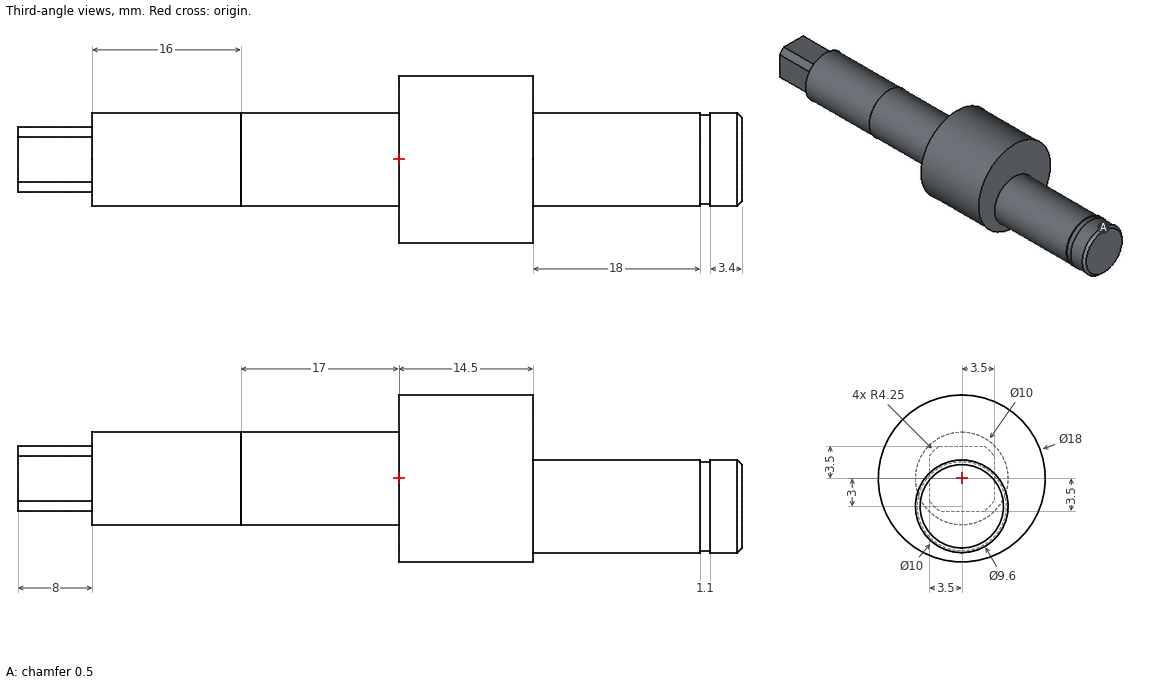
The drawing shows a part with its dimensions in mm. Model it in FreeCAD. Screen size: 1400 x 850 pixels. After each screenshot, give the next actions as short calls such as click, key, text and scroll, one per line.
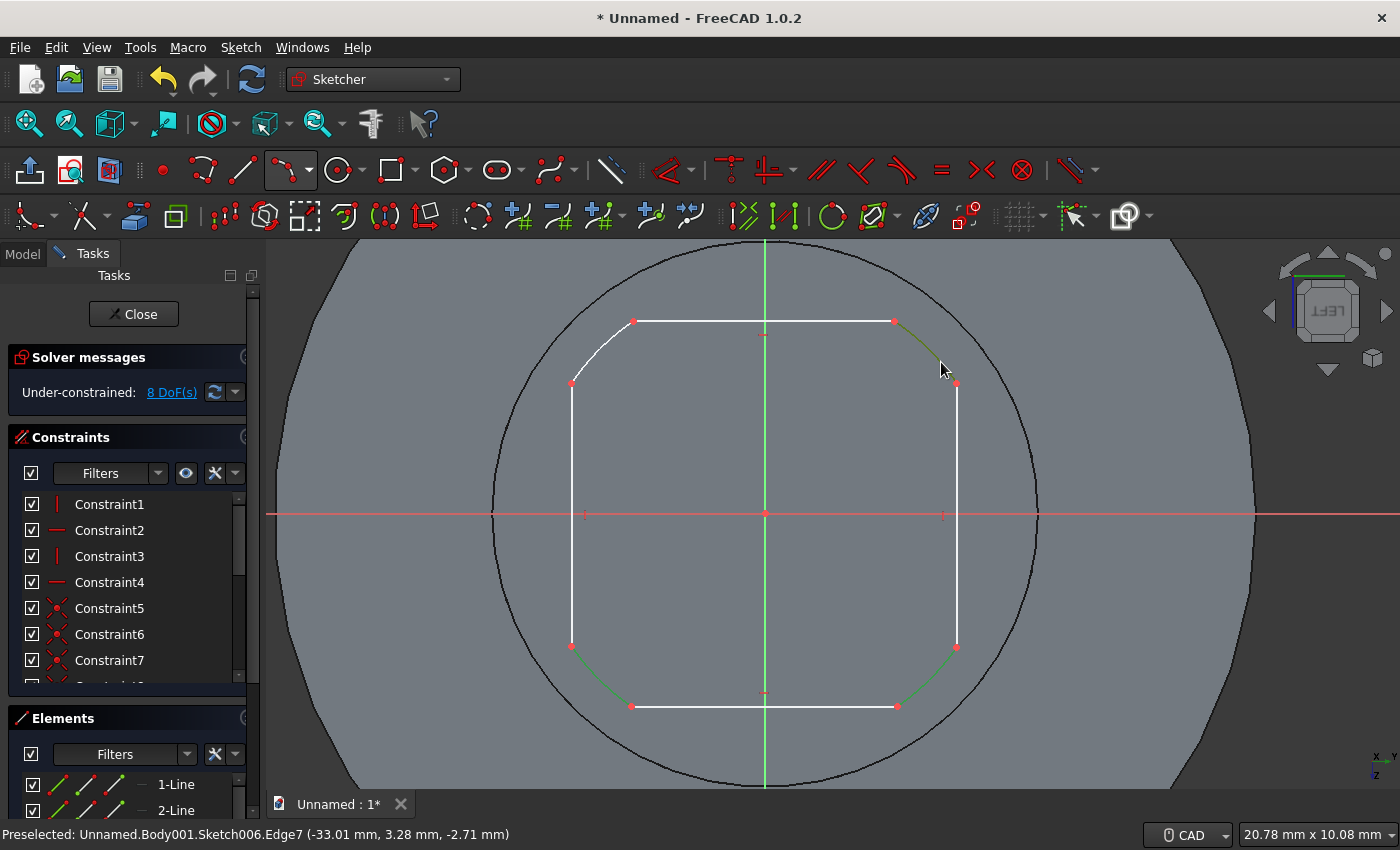
click(613, 337)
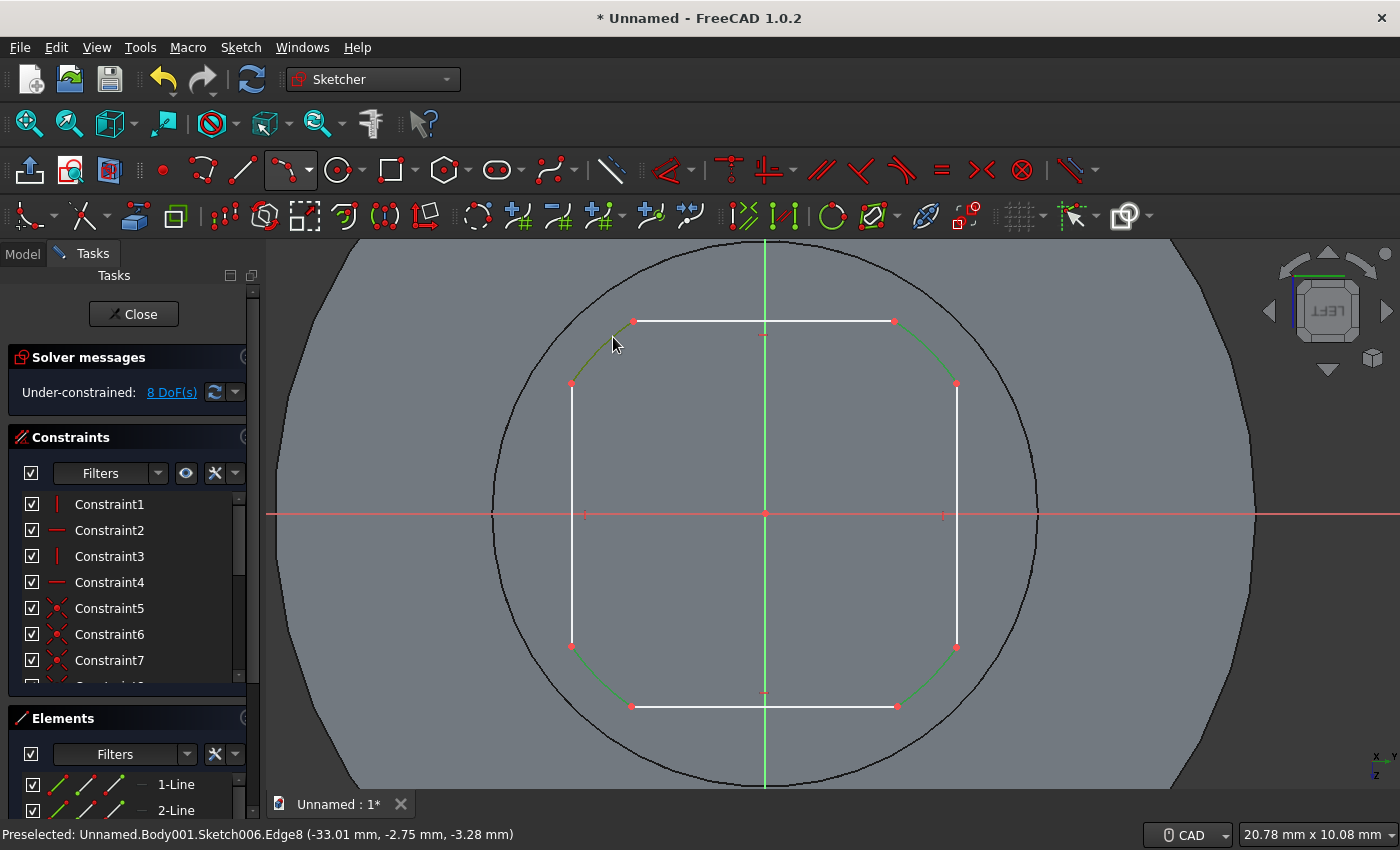
click(942, 170)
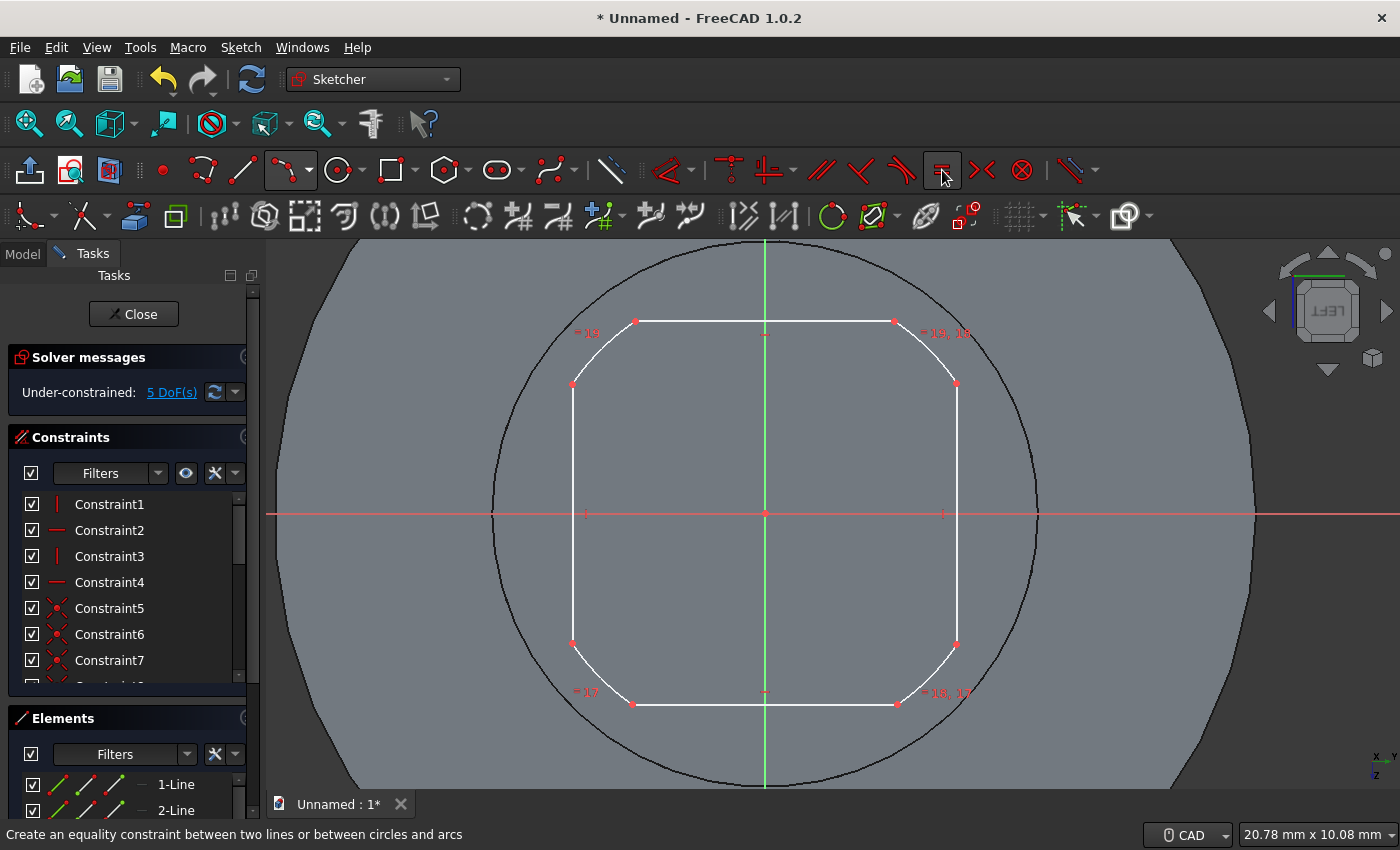
click(666, 170)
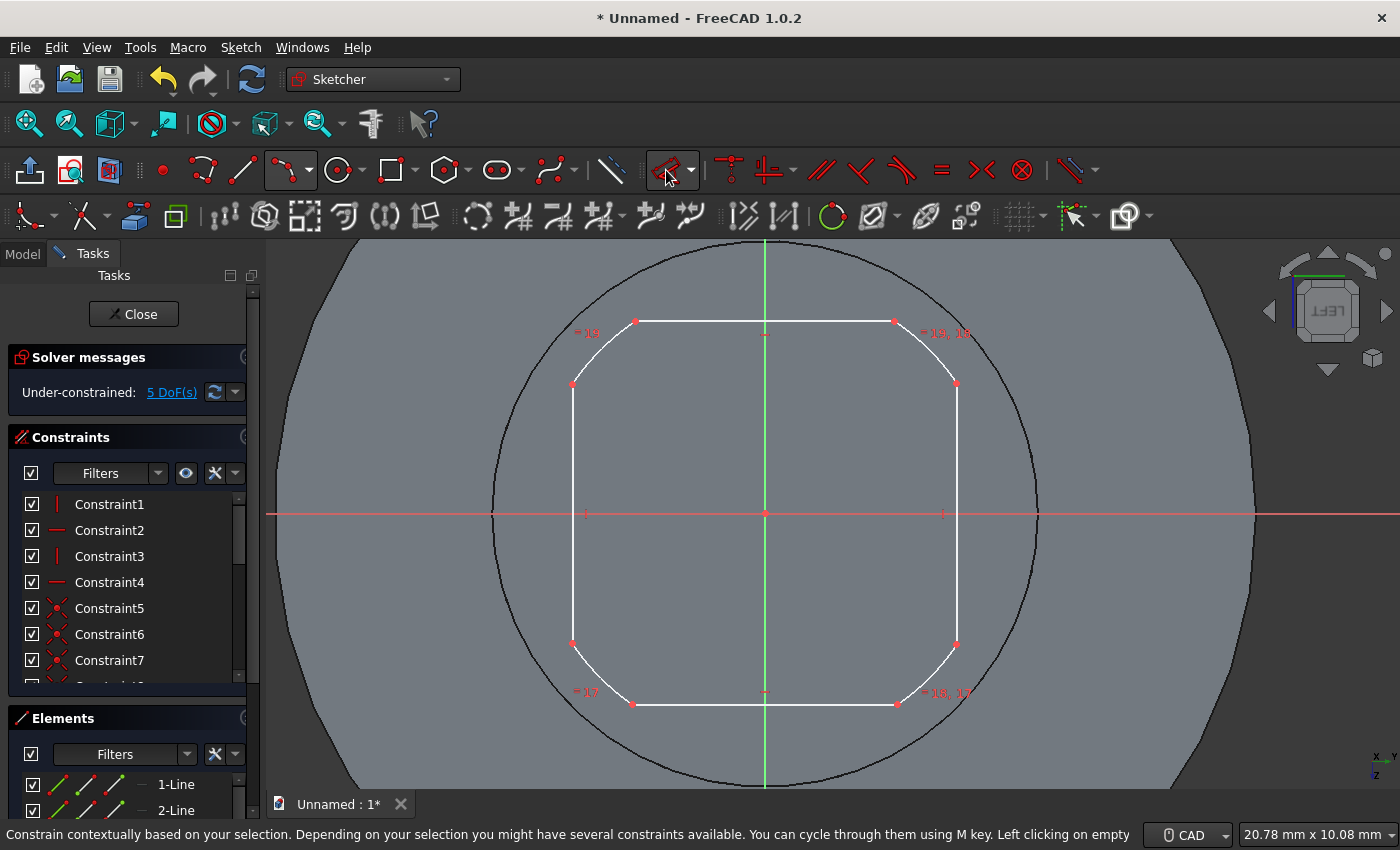
click(588, 665)
click(564, 686)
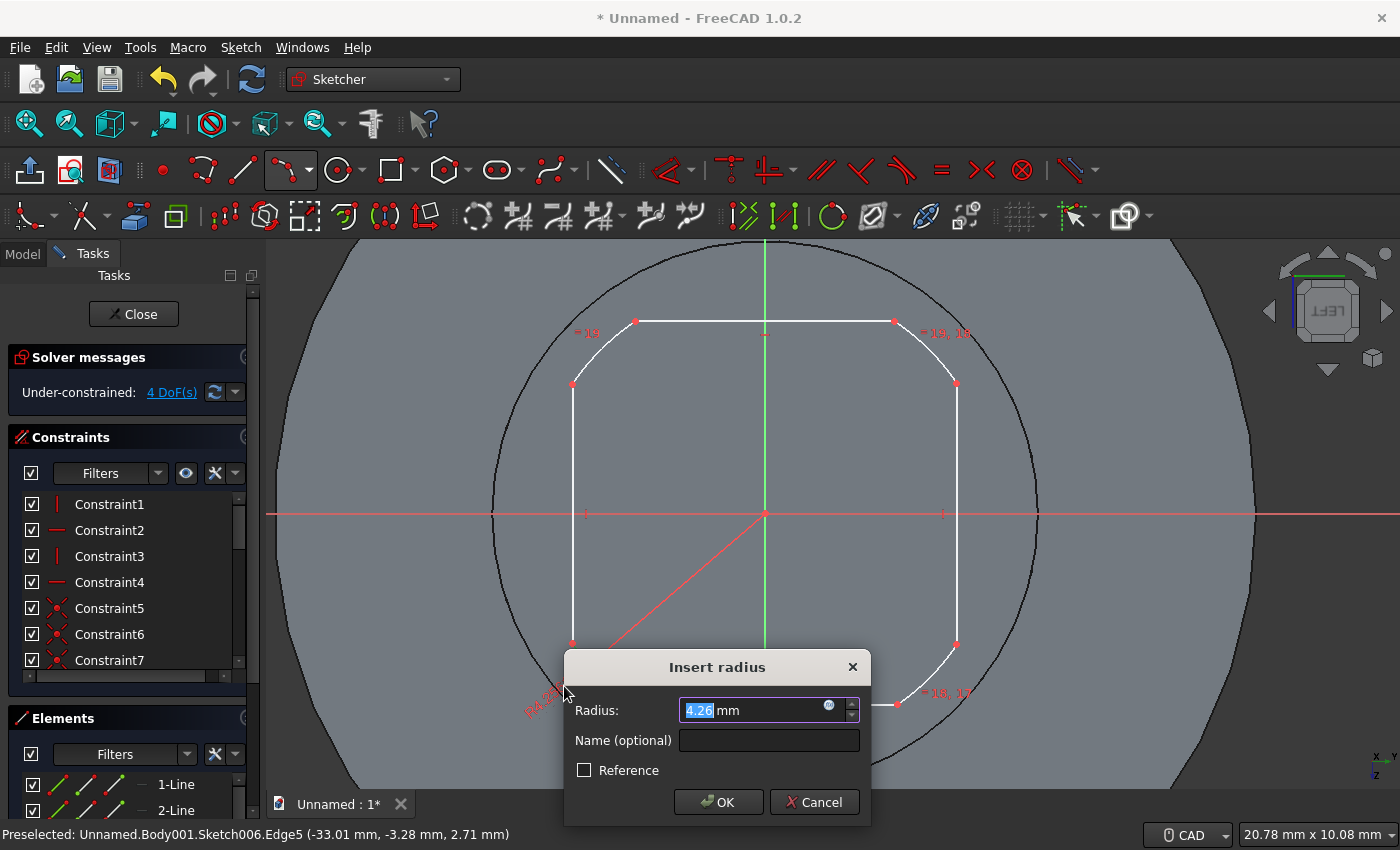
text(4.25)
key(Return)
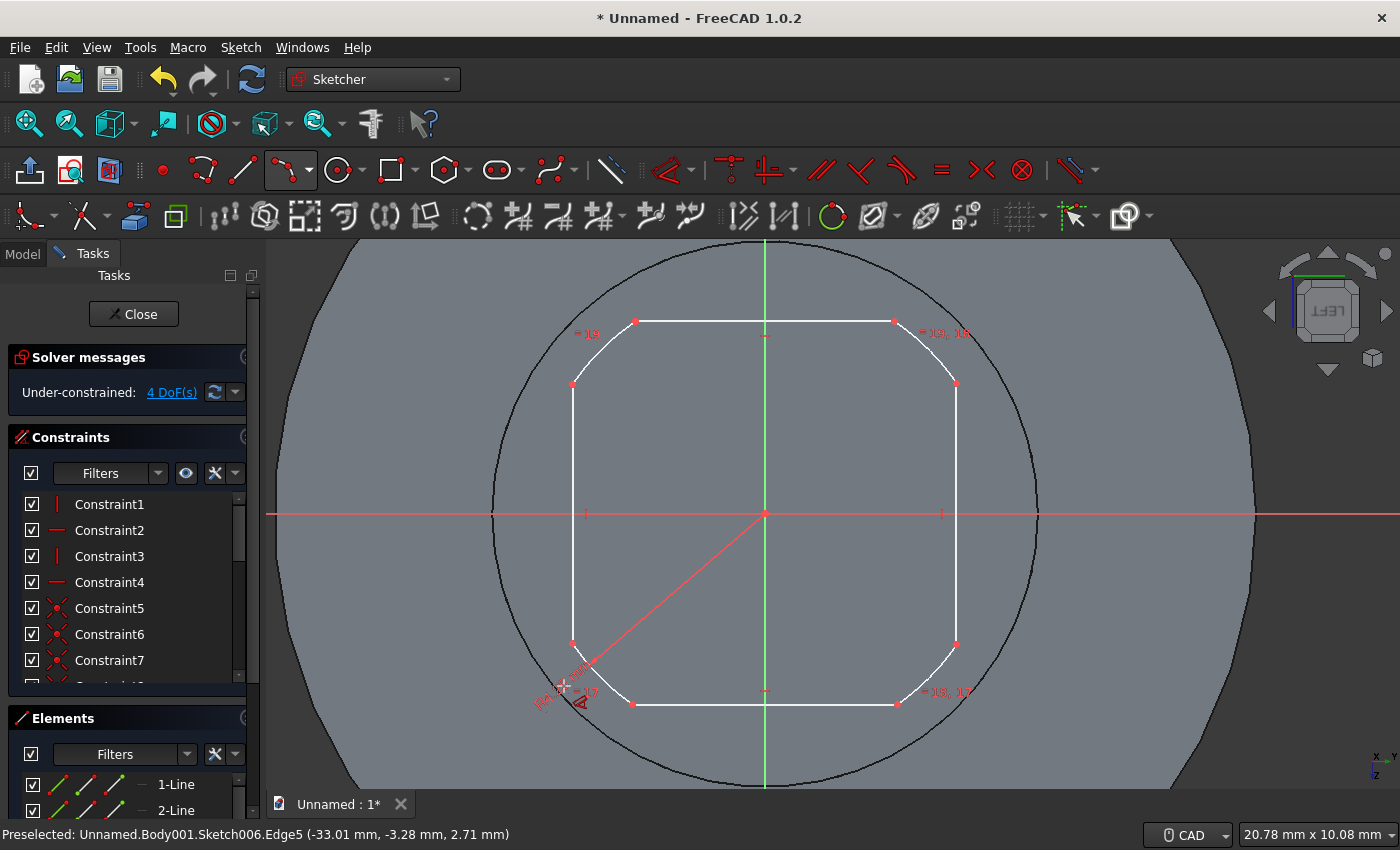
click(573, 384)
click(669, 350)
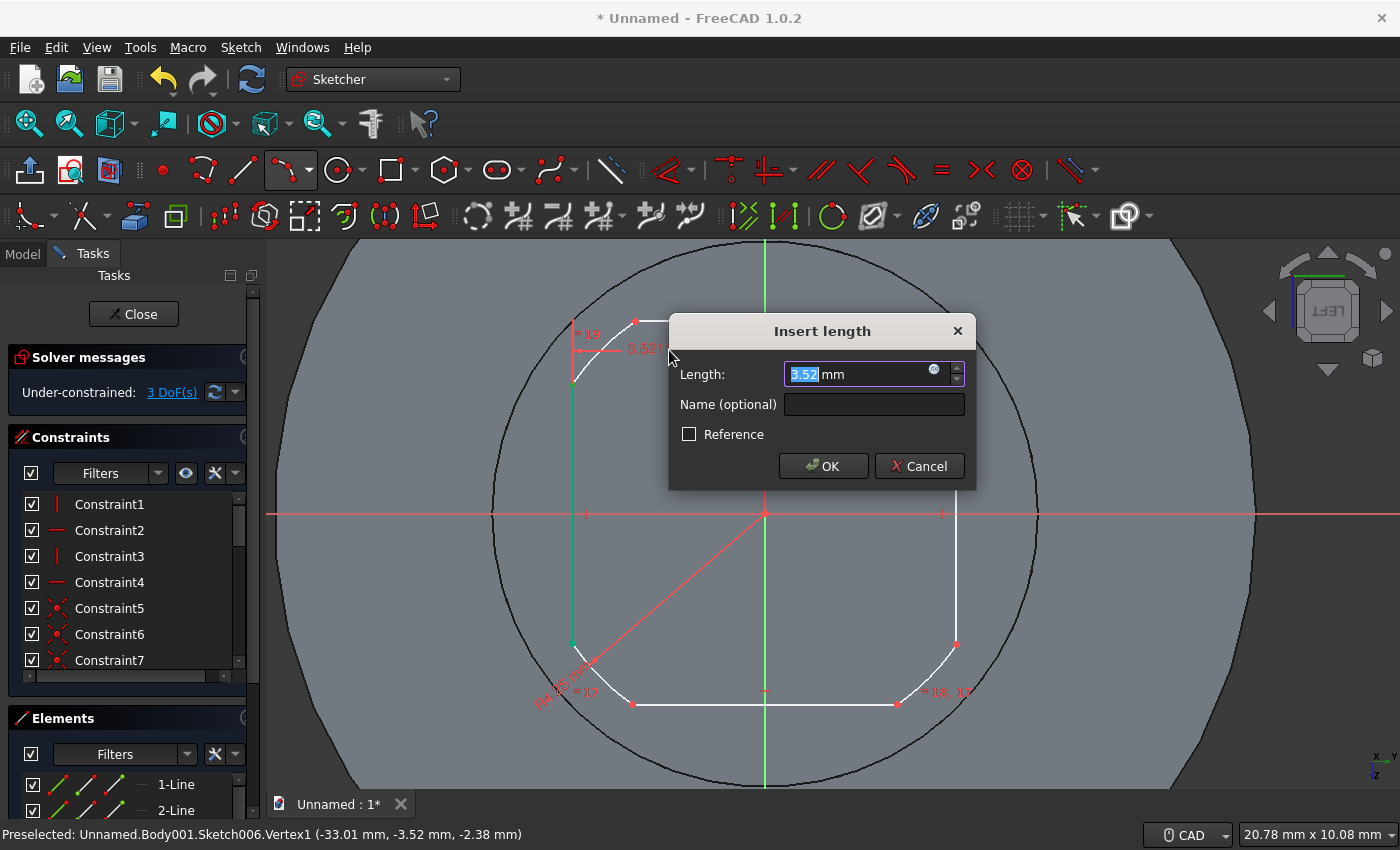
text(3.5)
key(Return)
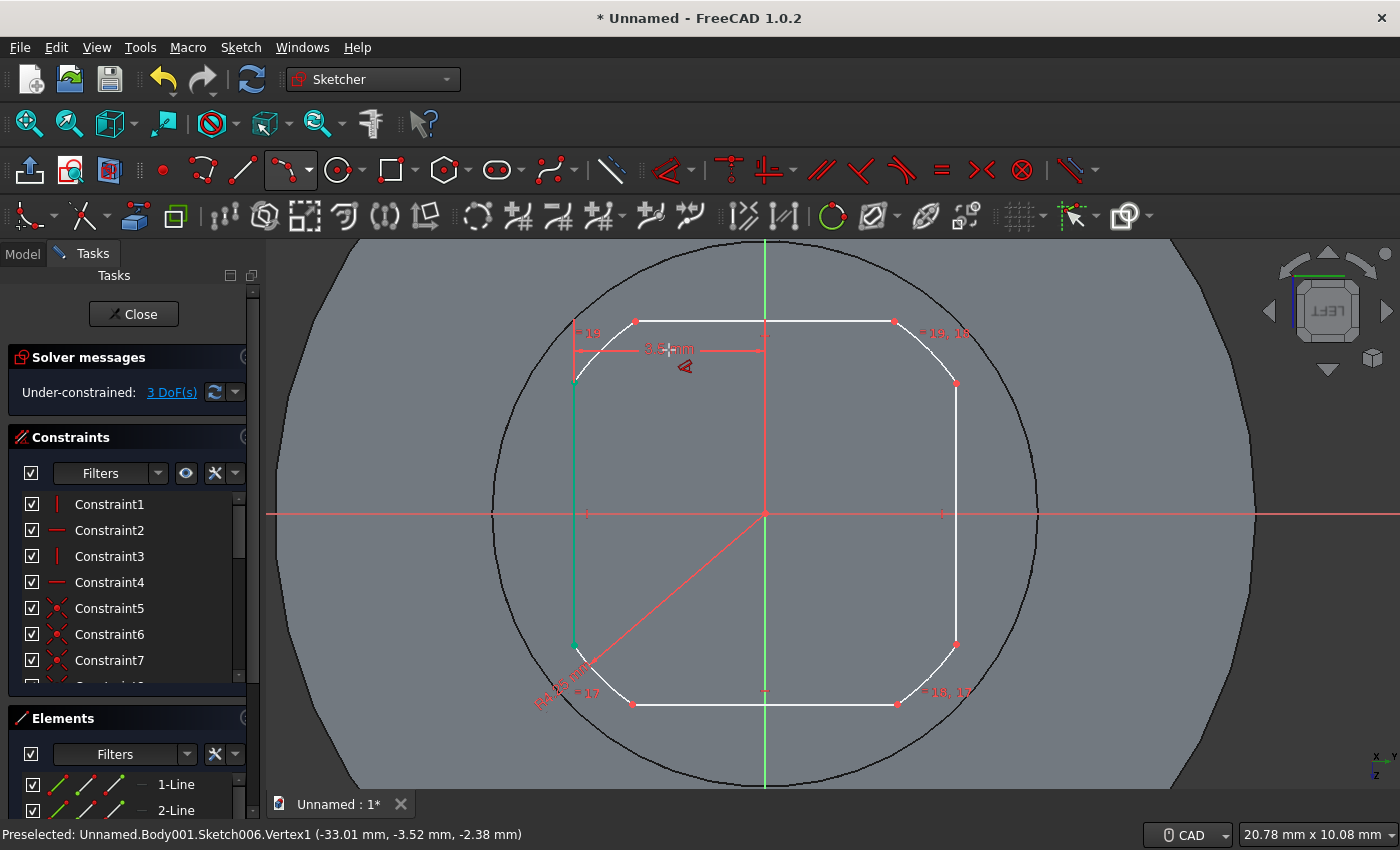
click(633, 705)
click(599, 609)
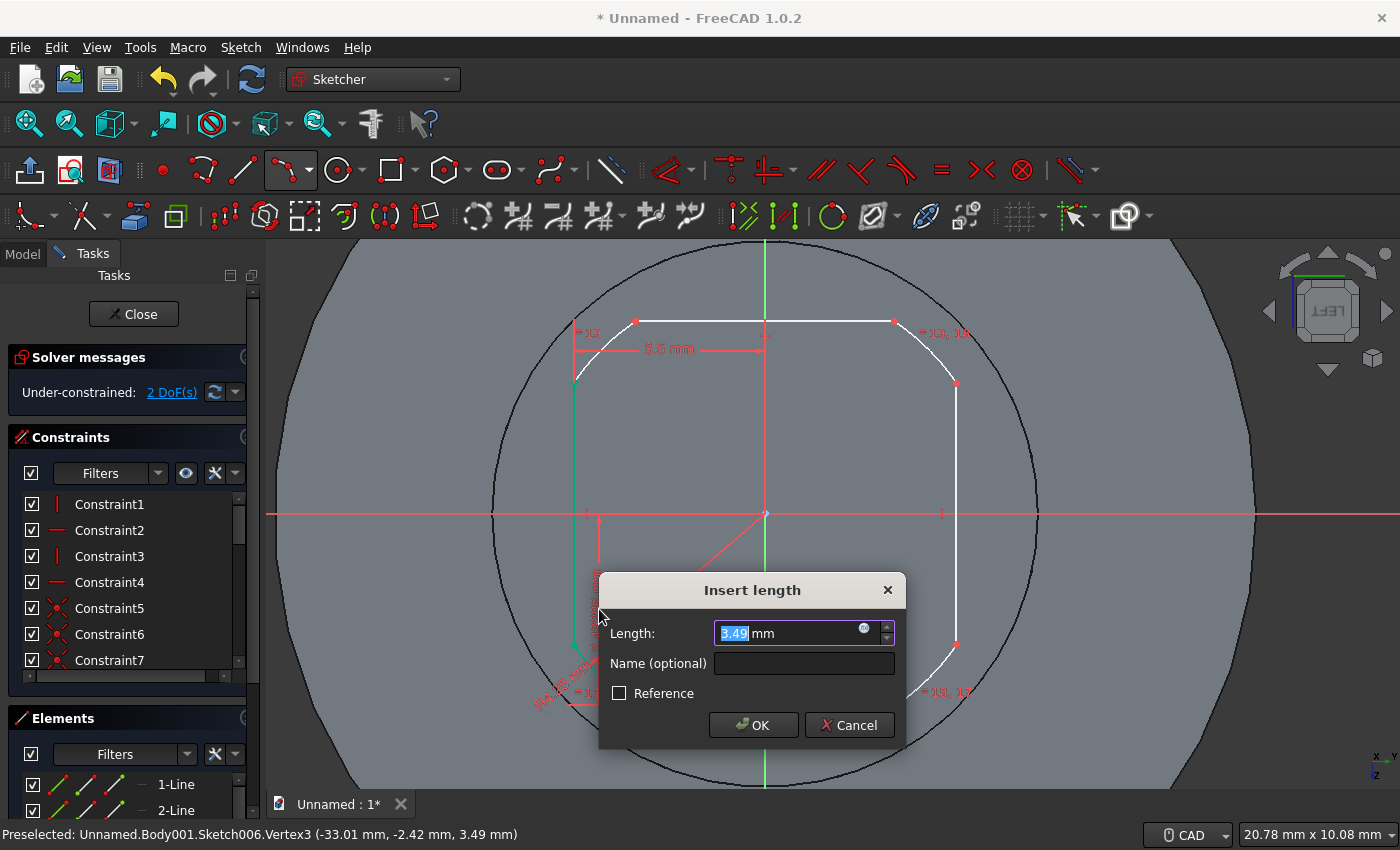
text(3.5)
key(Return)